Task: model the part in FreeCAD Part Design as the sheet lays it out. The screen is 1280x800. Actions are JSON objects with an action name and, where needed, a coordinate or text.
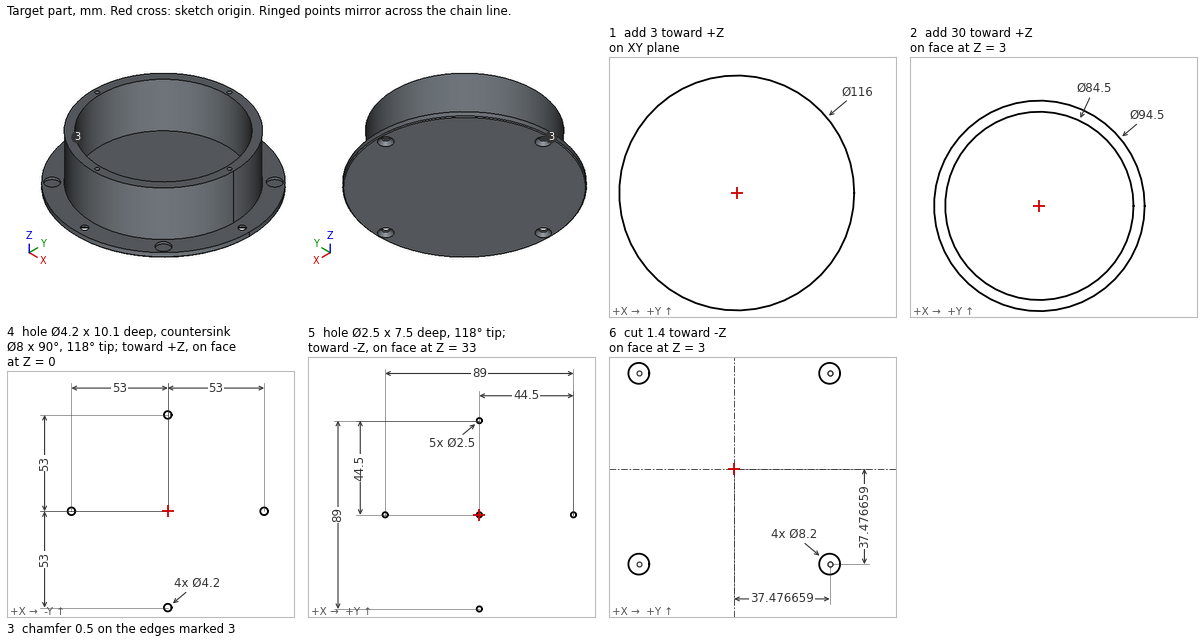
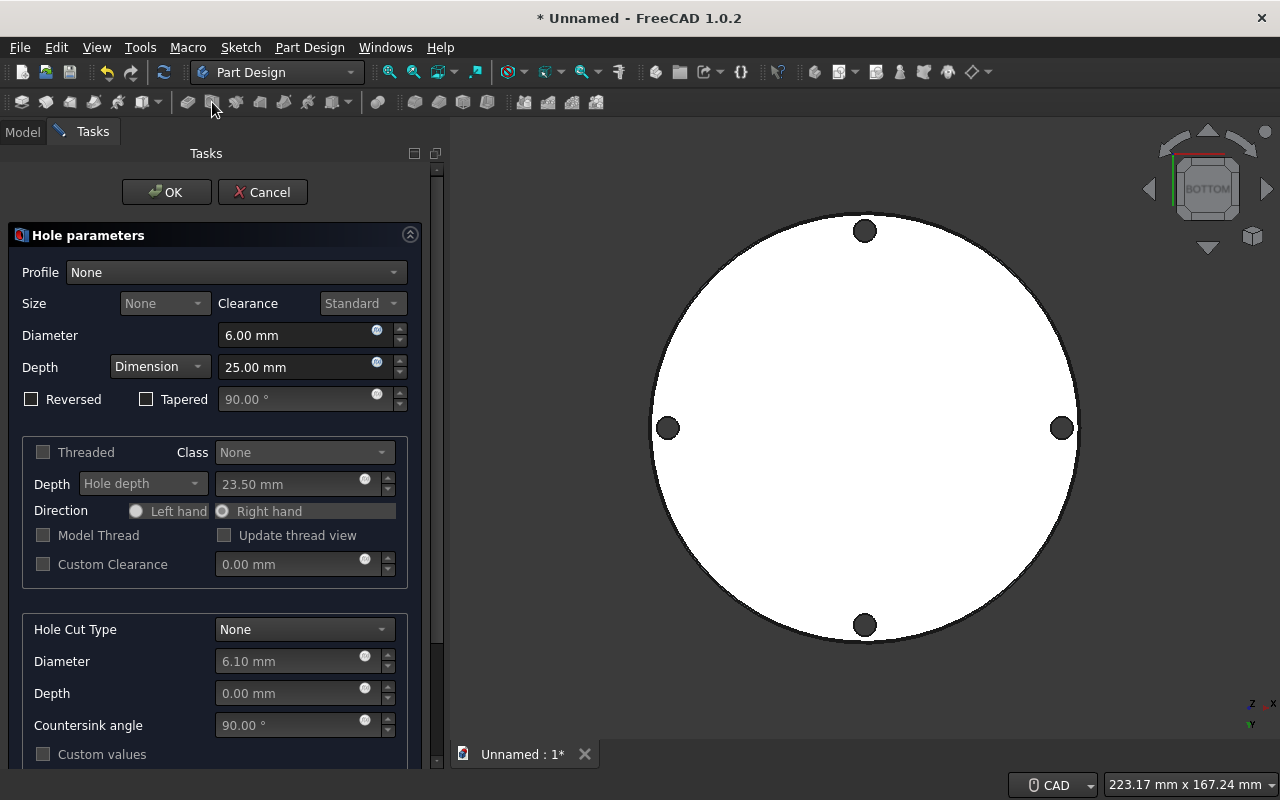
{"action": "triple_click", "coordinate": [305, 335]}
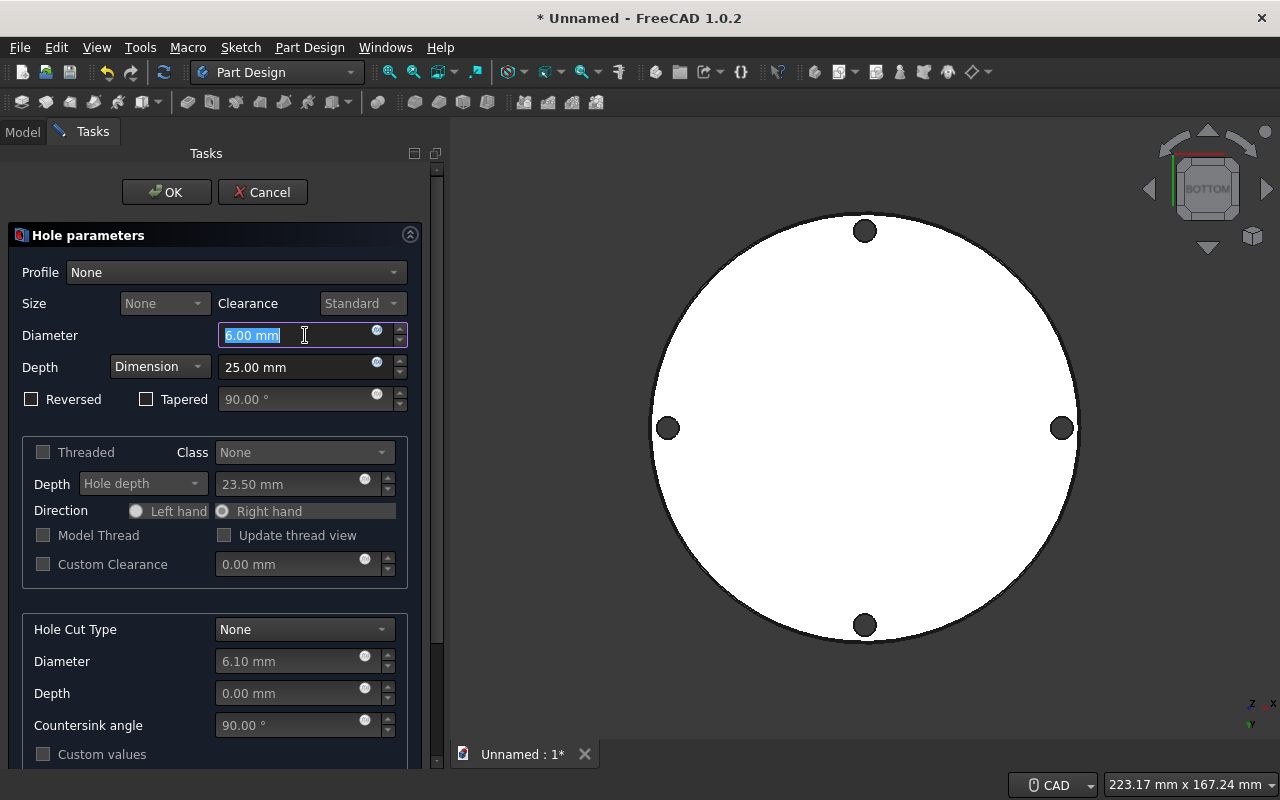
{"action": "type", "text": "4.2"}
{"action": "key", "text": "Tab"}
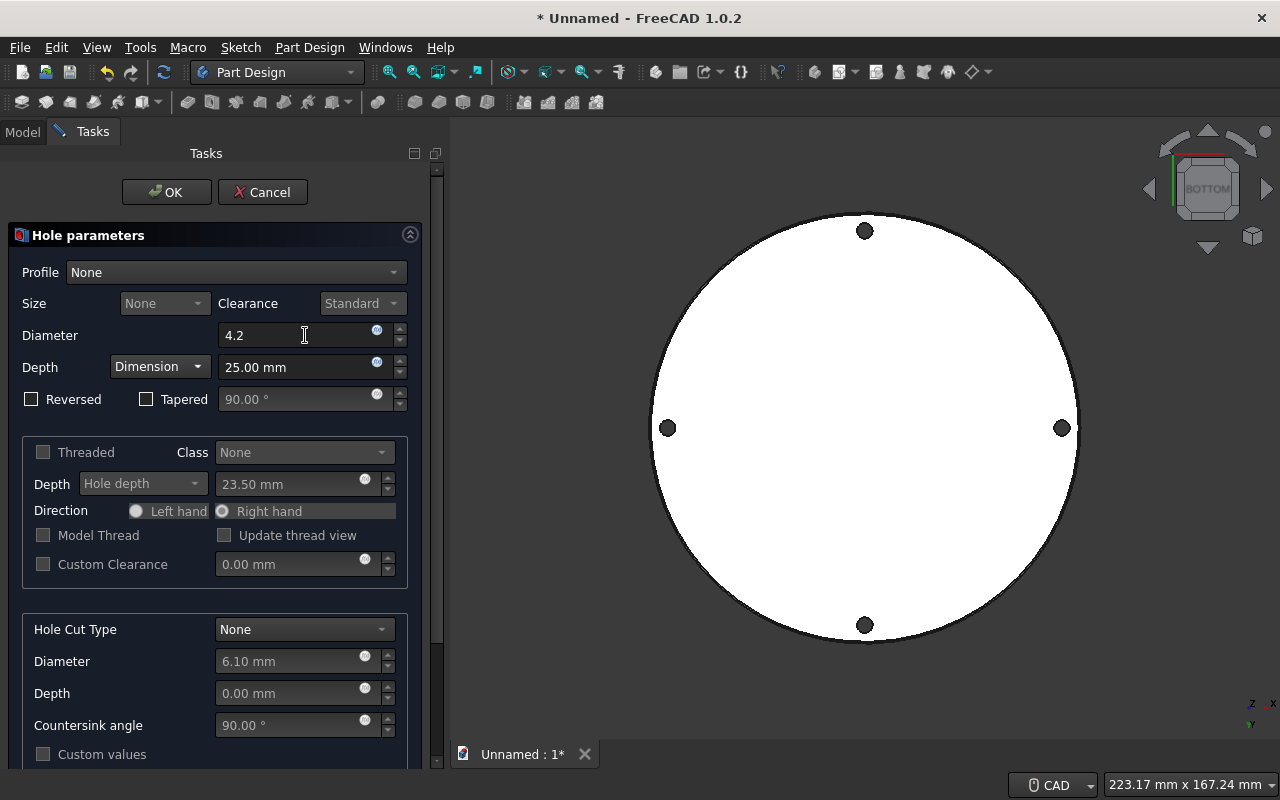
{"action": "triple_click", "coordinate": [305, 367]}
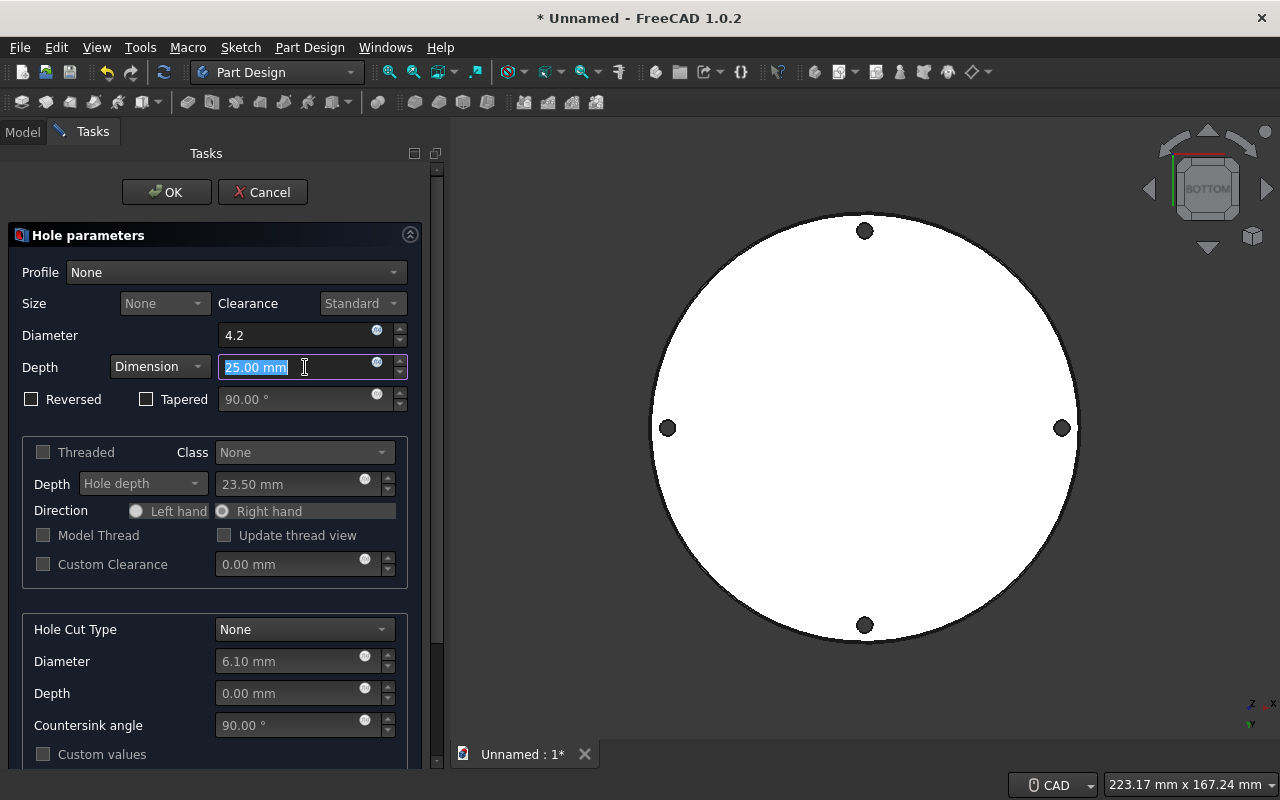
{"action": "type", "text": "10.1"}
{"action": "key", "text": "Tab"}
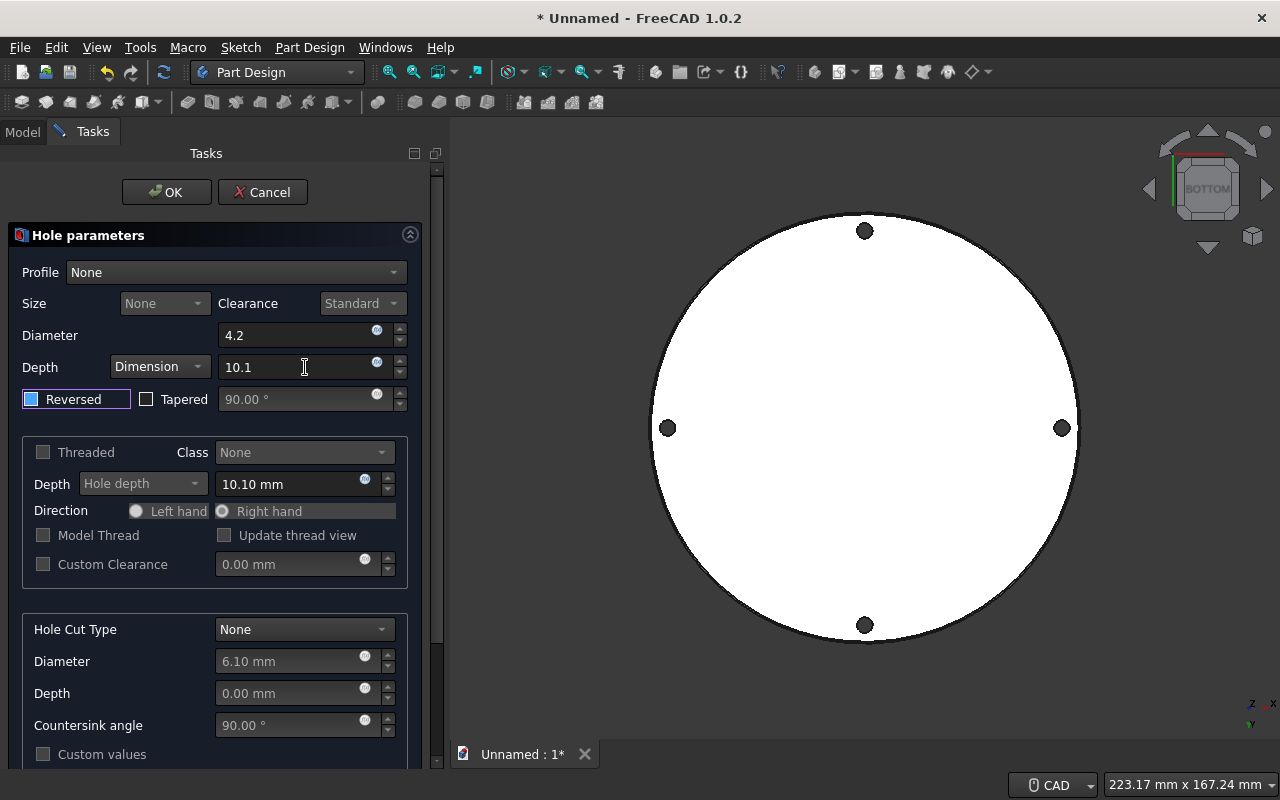
{"action": "left_click", "coordinate": [306, 630]}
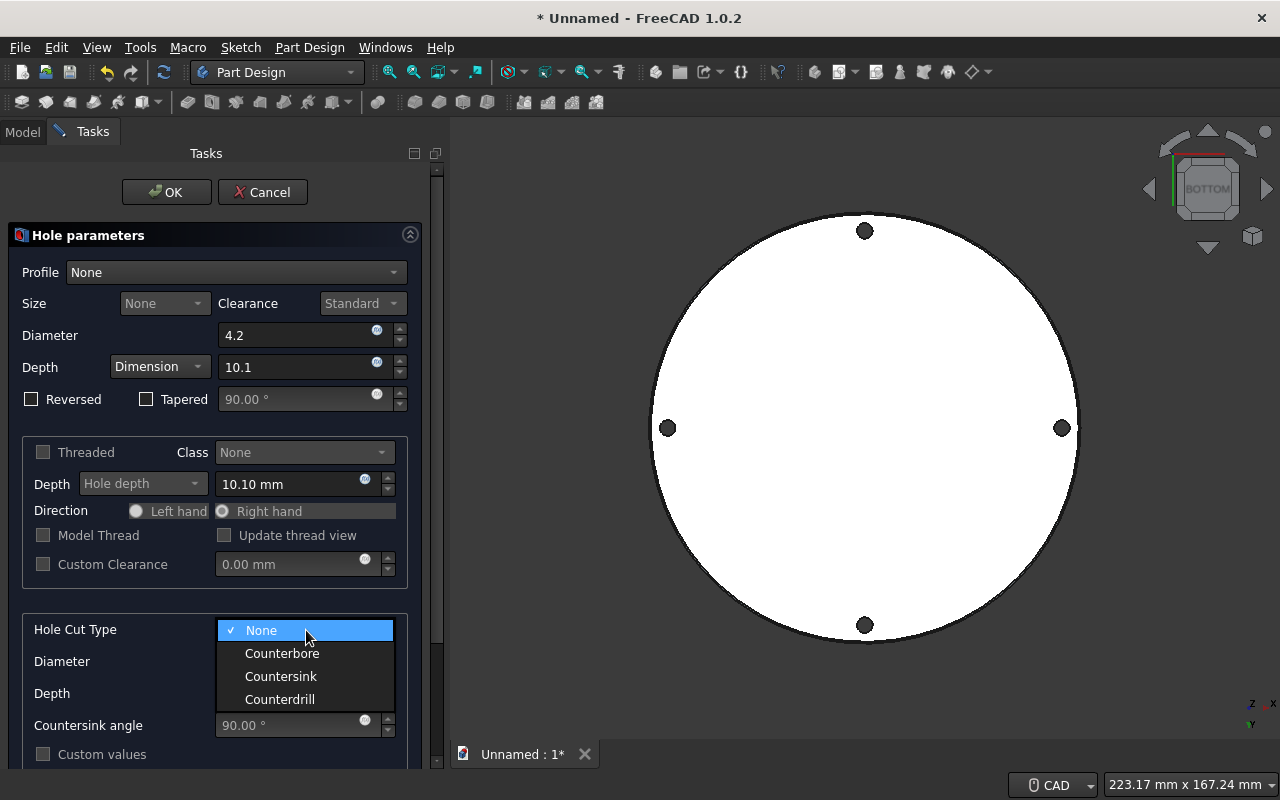
{"action": "left_click", "coordinate": [304, 676]}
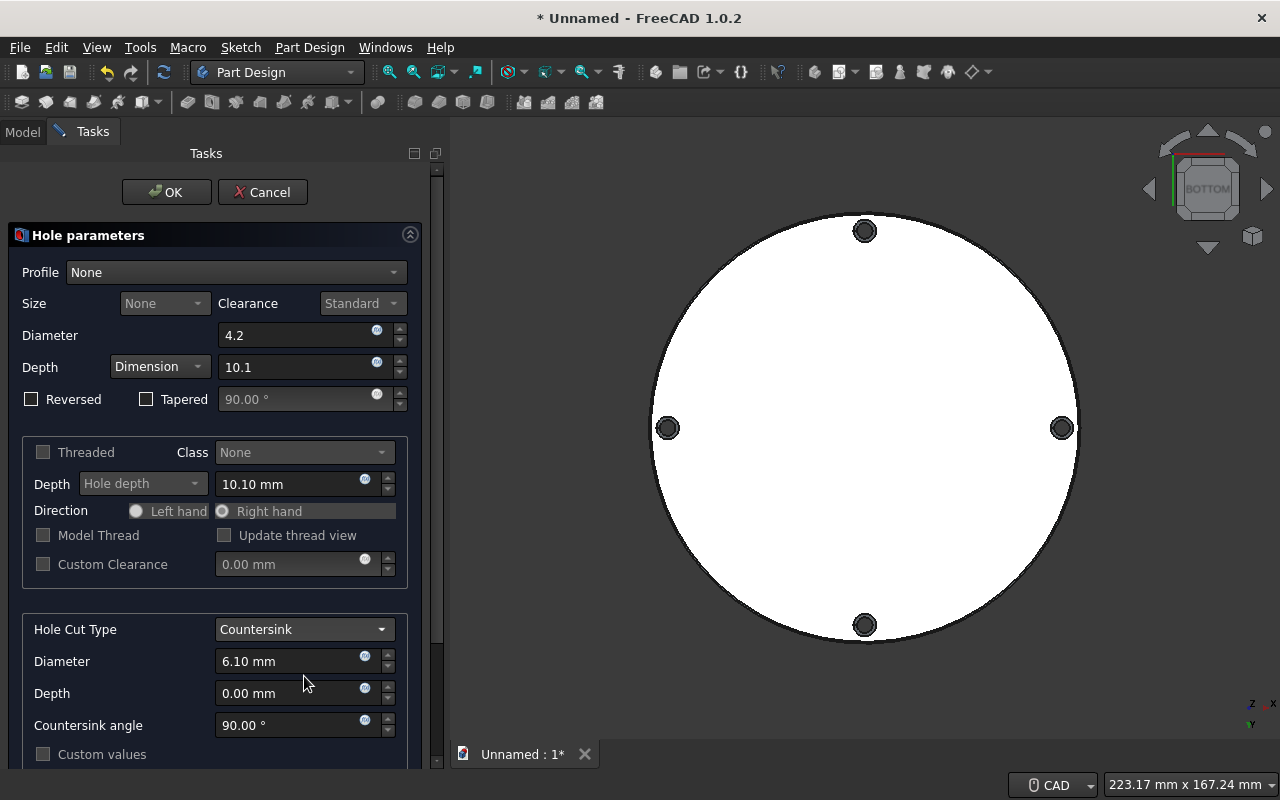
{"action": "triple_click", "coordinate": [298, 661]}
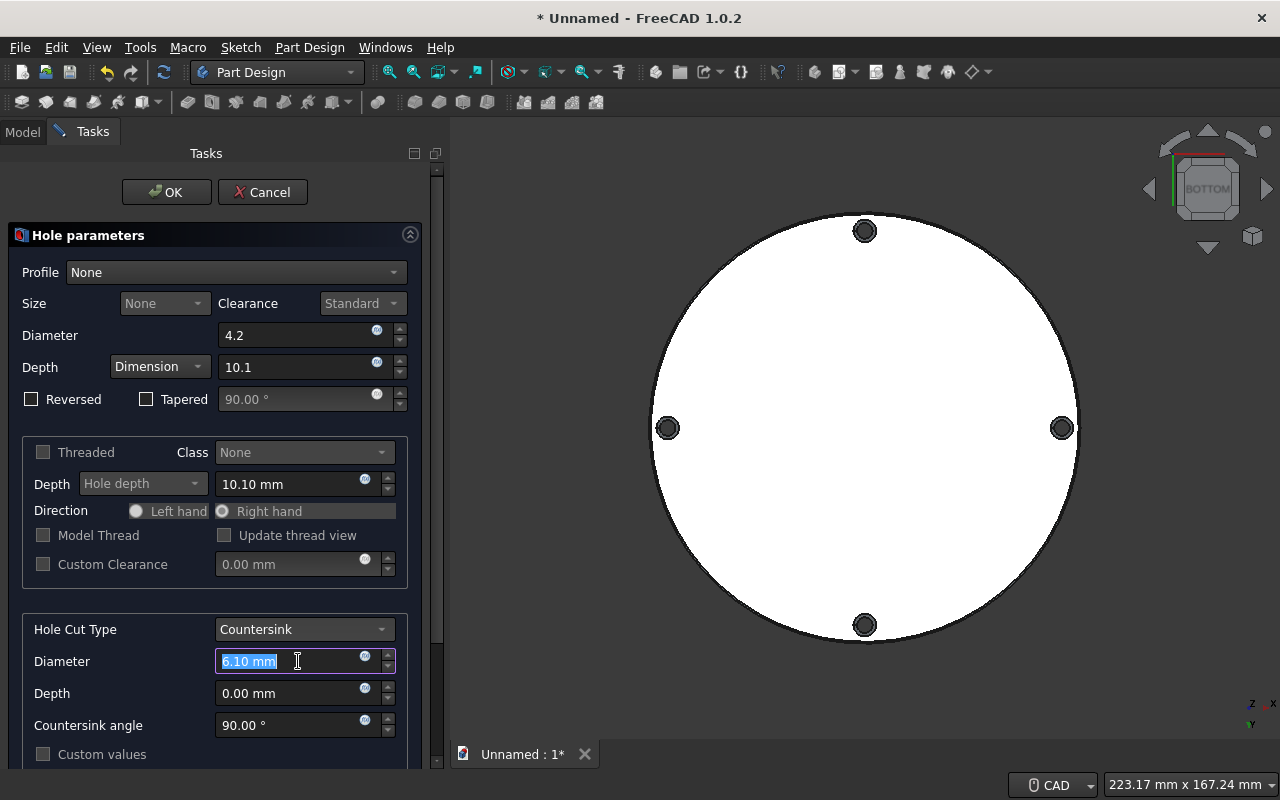
{"action": "type", "text": "8"}
{"action": "key", "text": "Tab"}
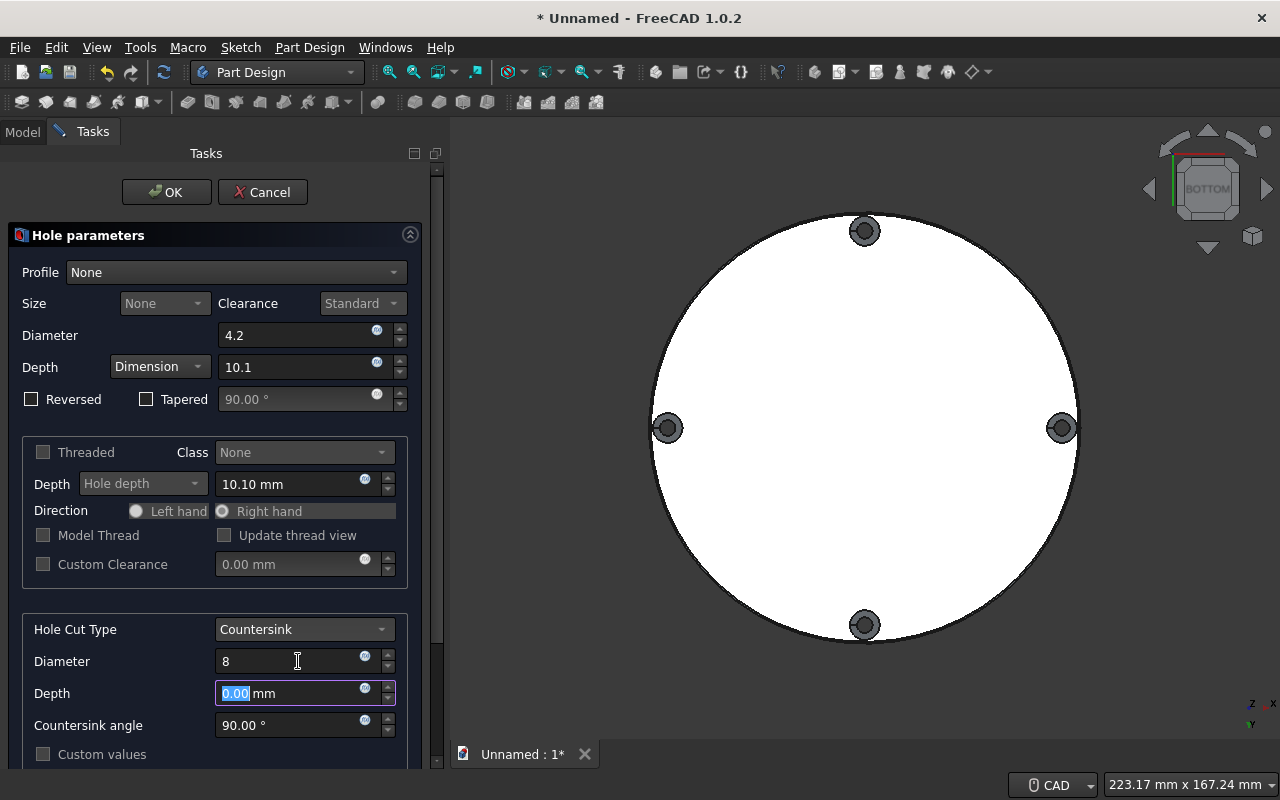
{"action": "left_click", "coordinate": [167, 192]}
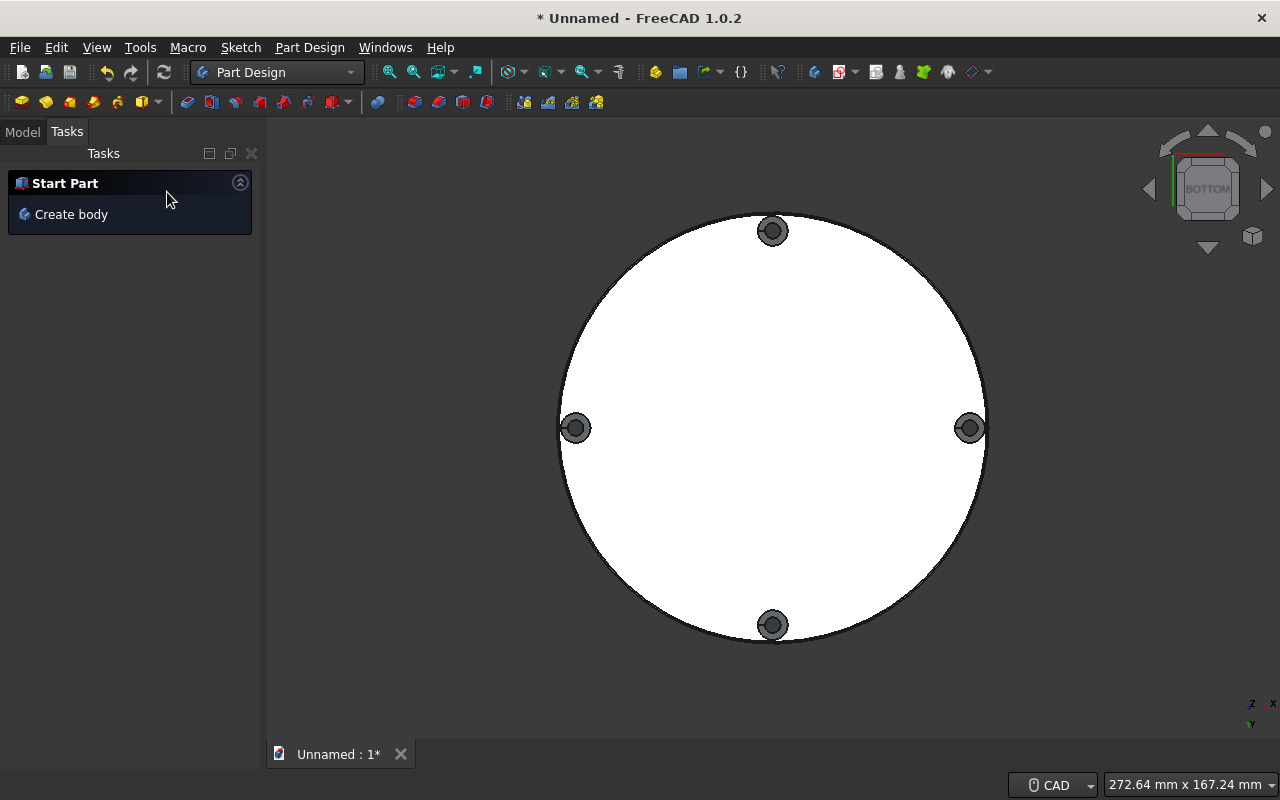
{"action": "key", "text": "0"}